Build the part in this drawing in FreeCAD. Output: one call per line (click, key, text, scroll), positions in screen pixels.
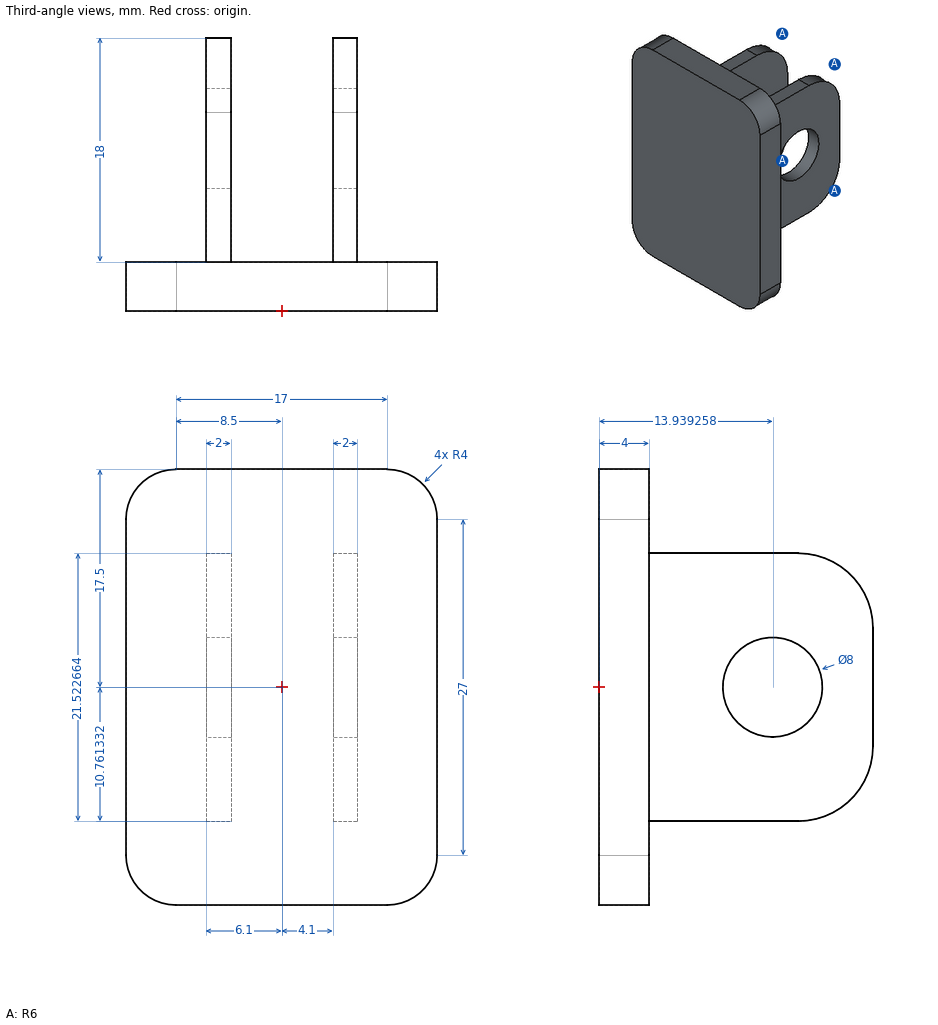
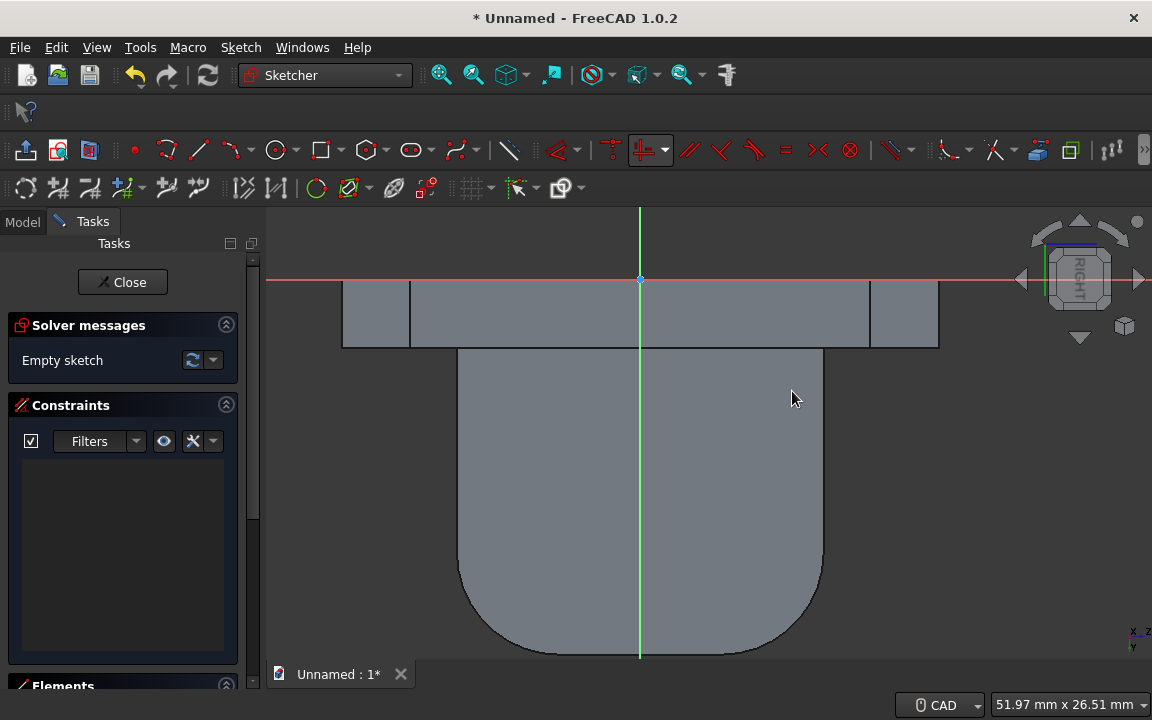
click(276, 150)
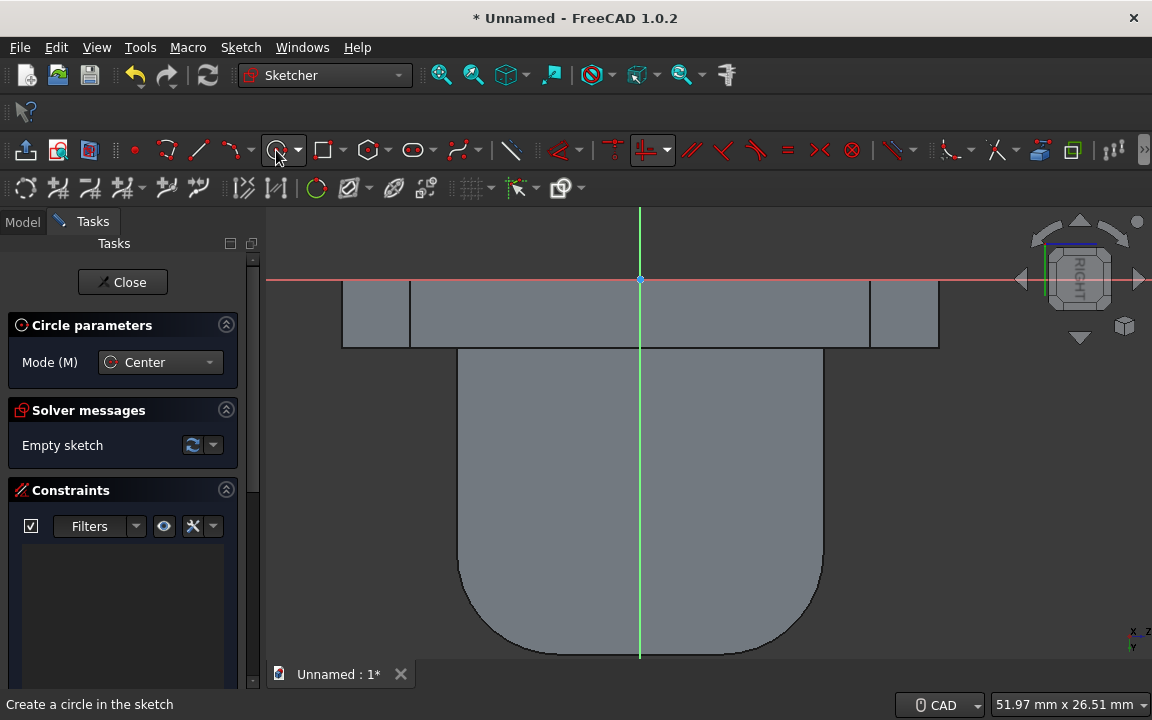
click(640, 517)
move(688, 469)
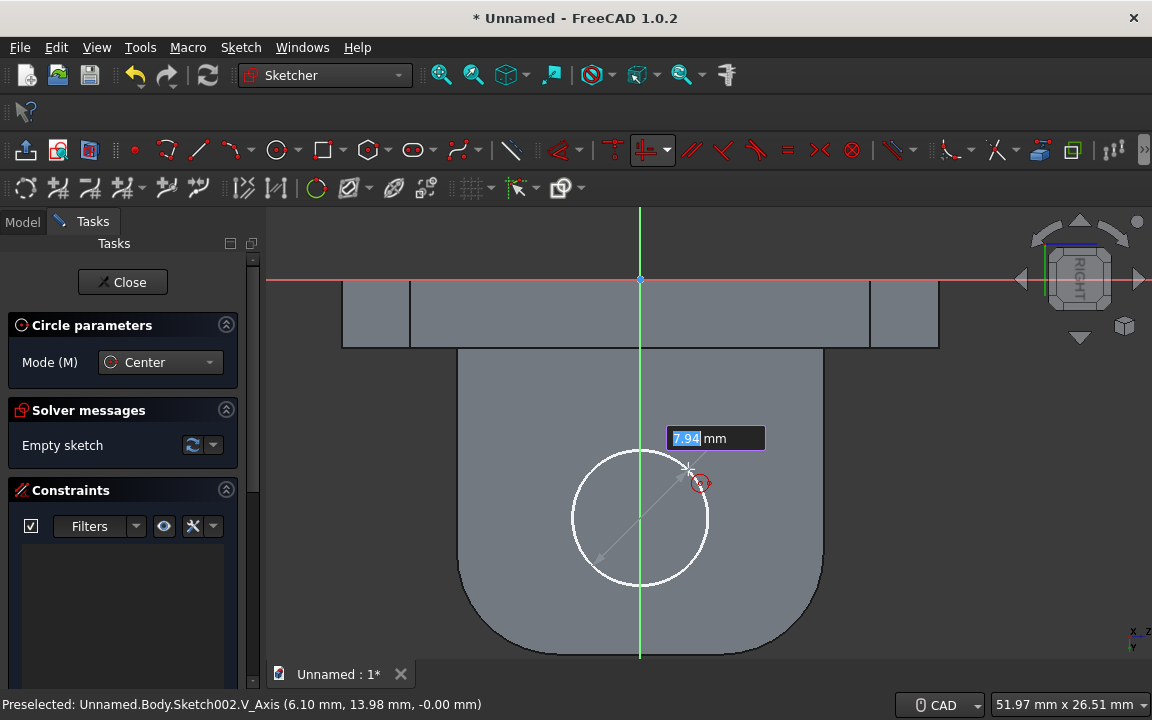
text(8)
key(Return)
key(Escape)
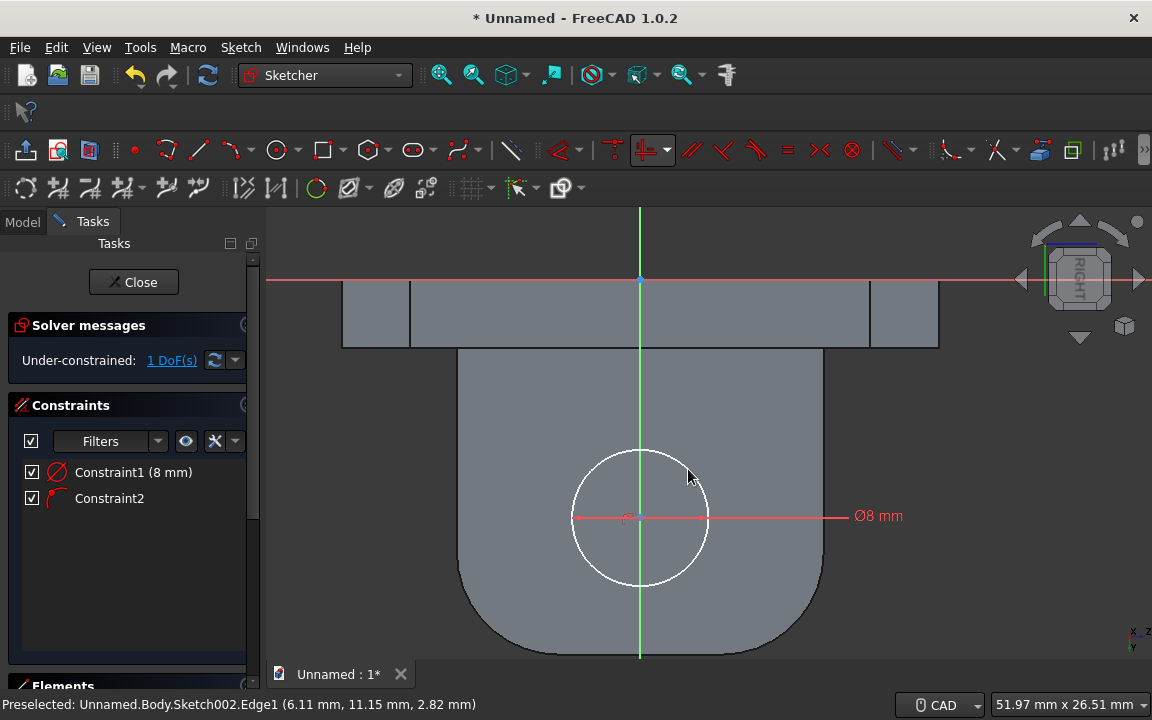
click(558, 150)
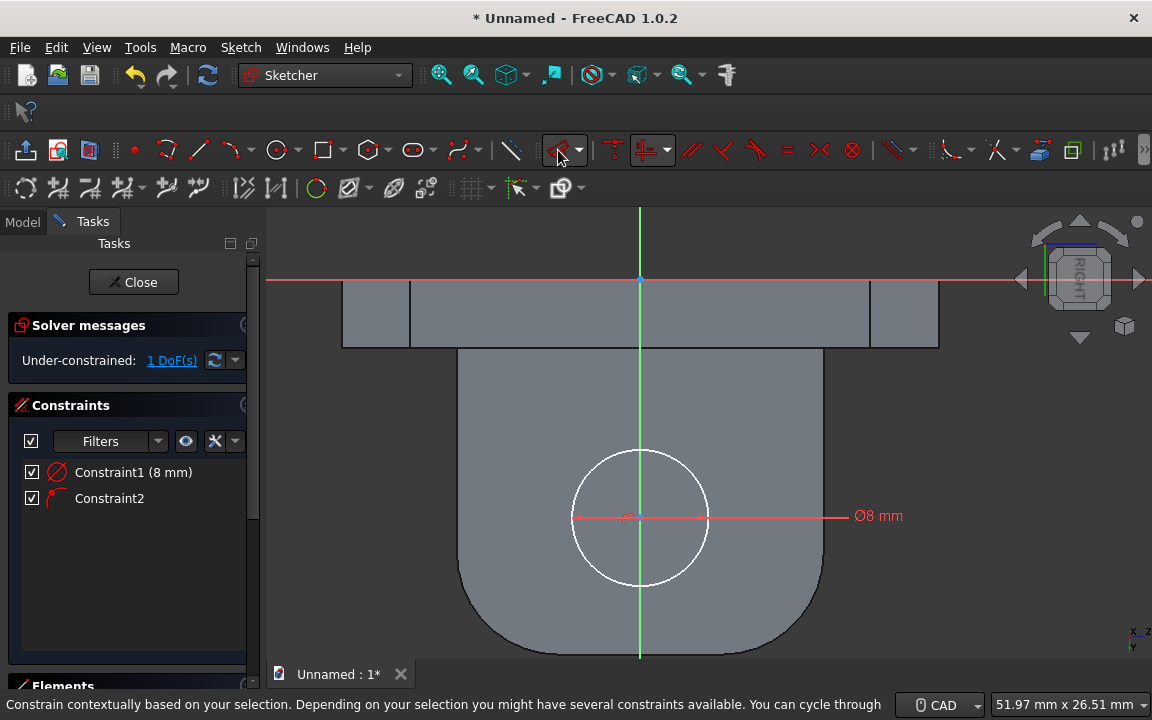
click(640, 518)
click(674, 399)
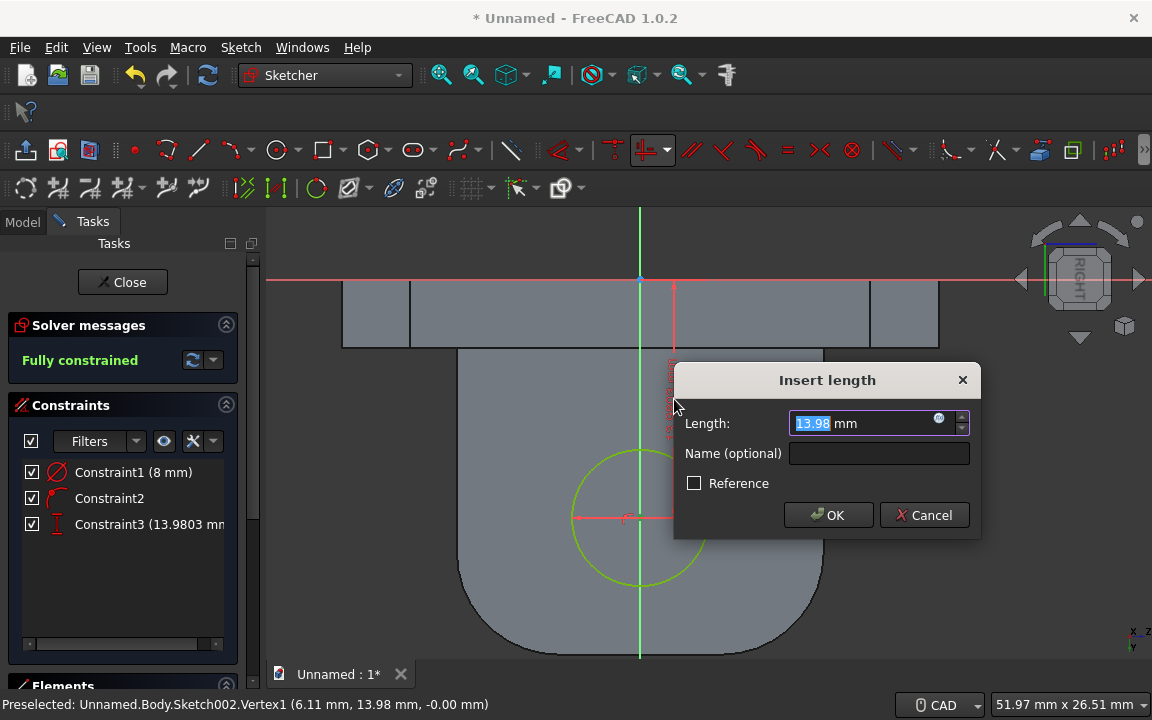
text(13.939258)
key(Return)
key(Escape)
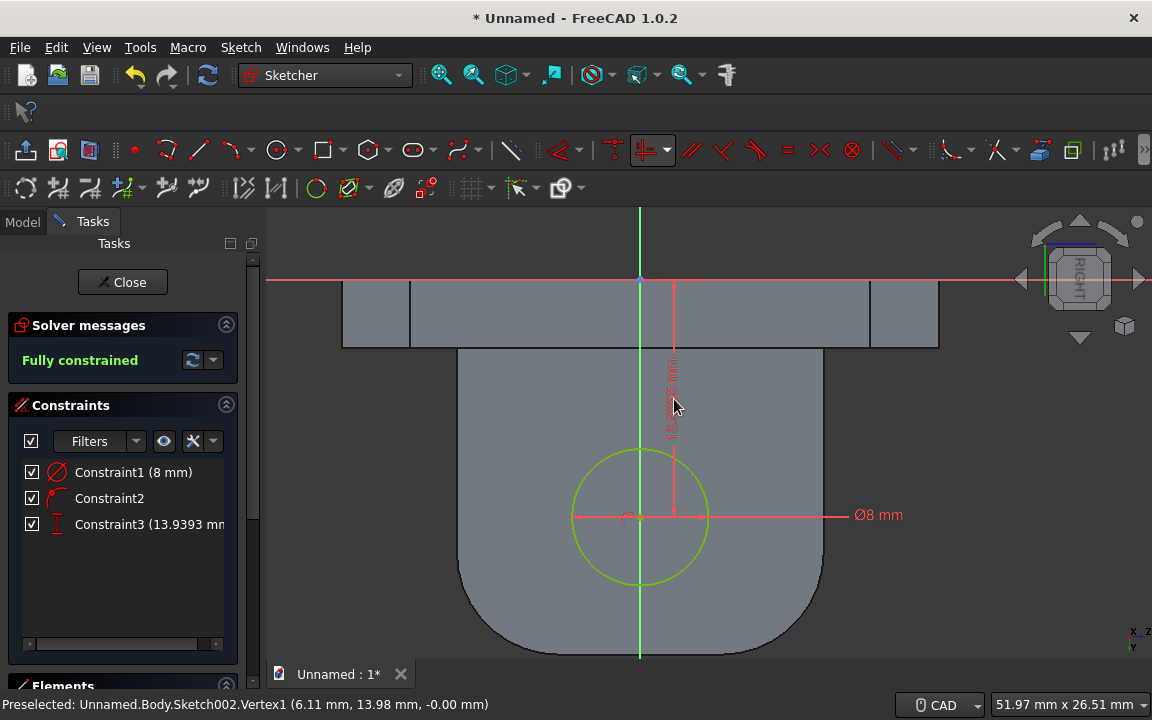
click(123, 282)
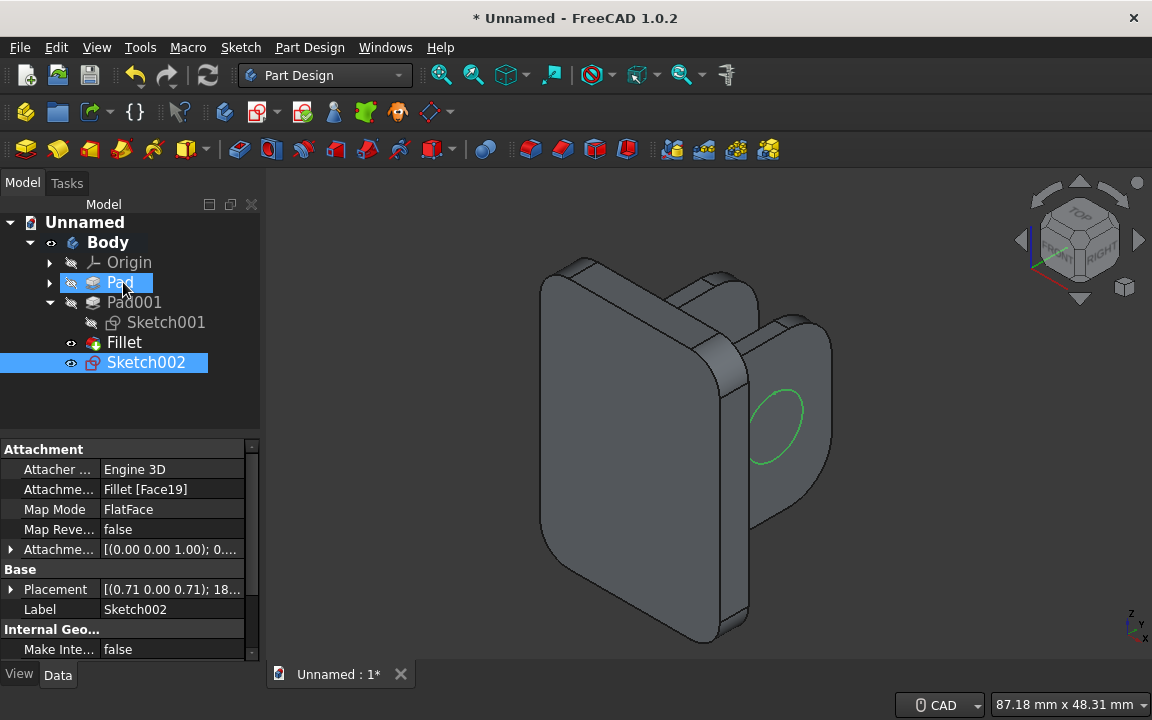
click(240, 150)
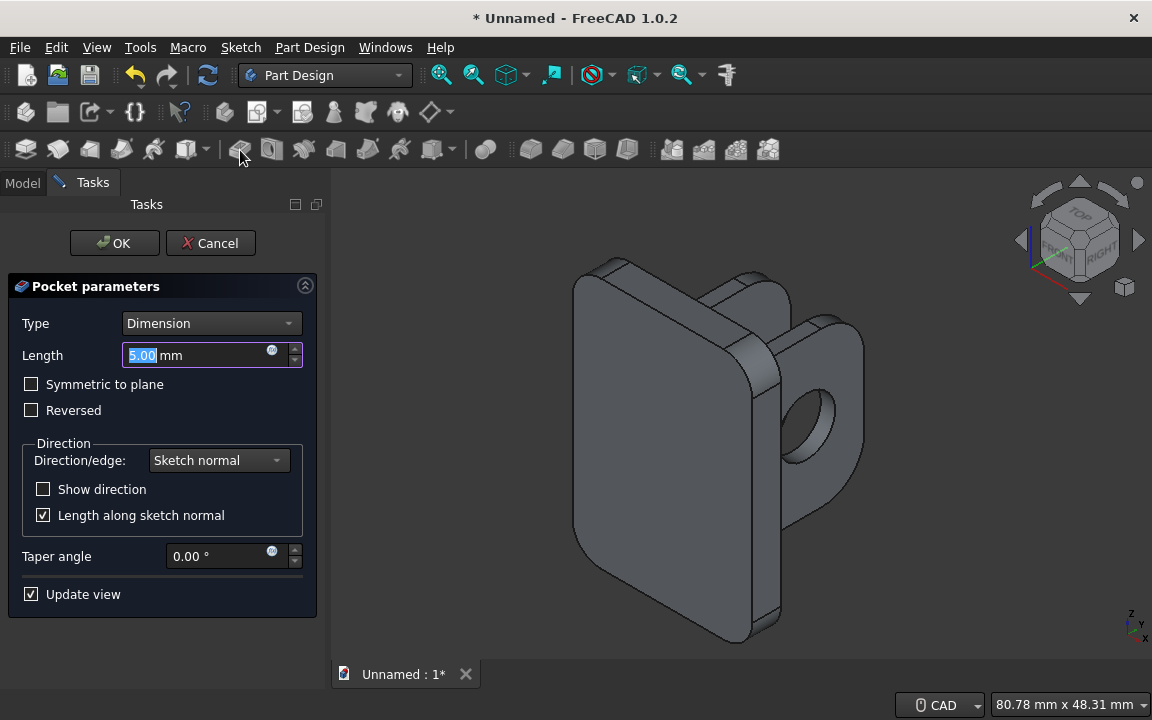
click(212, 324)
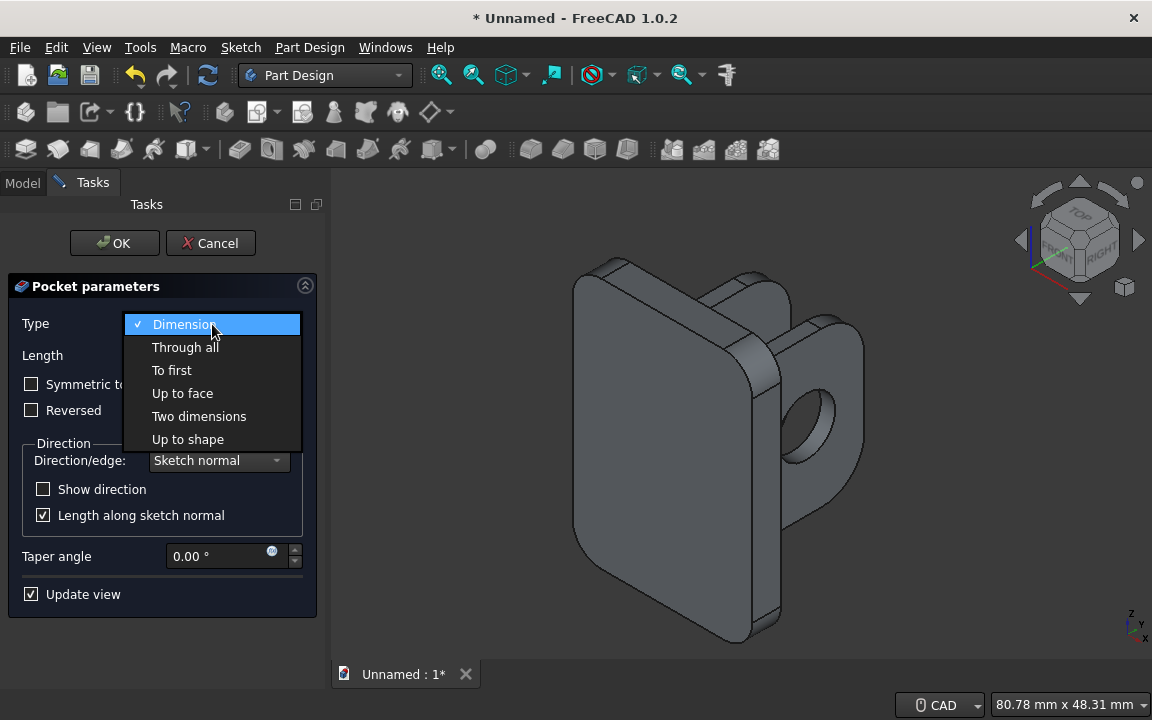
click(212, 348)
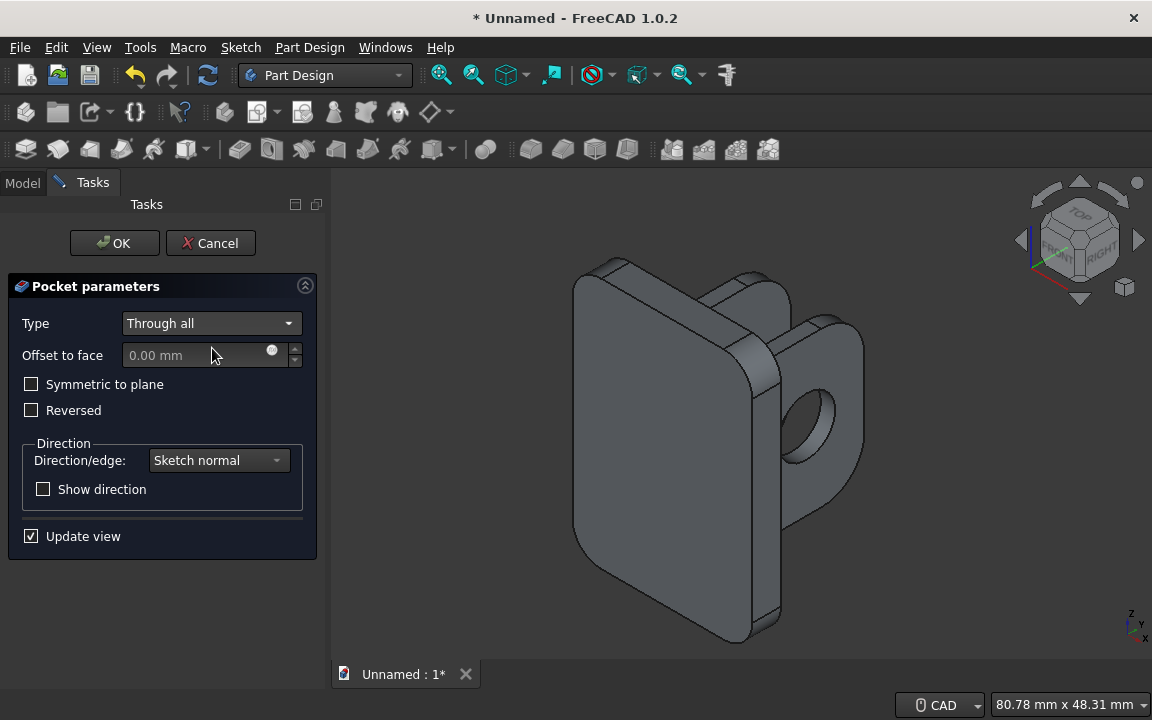
click(115, 243)